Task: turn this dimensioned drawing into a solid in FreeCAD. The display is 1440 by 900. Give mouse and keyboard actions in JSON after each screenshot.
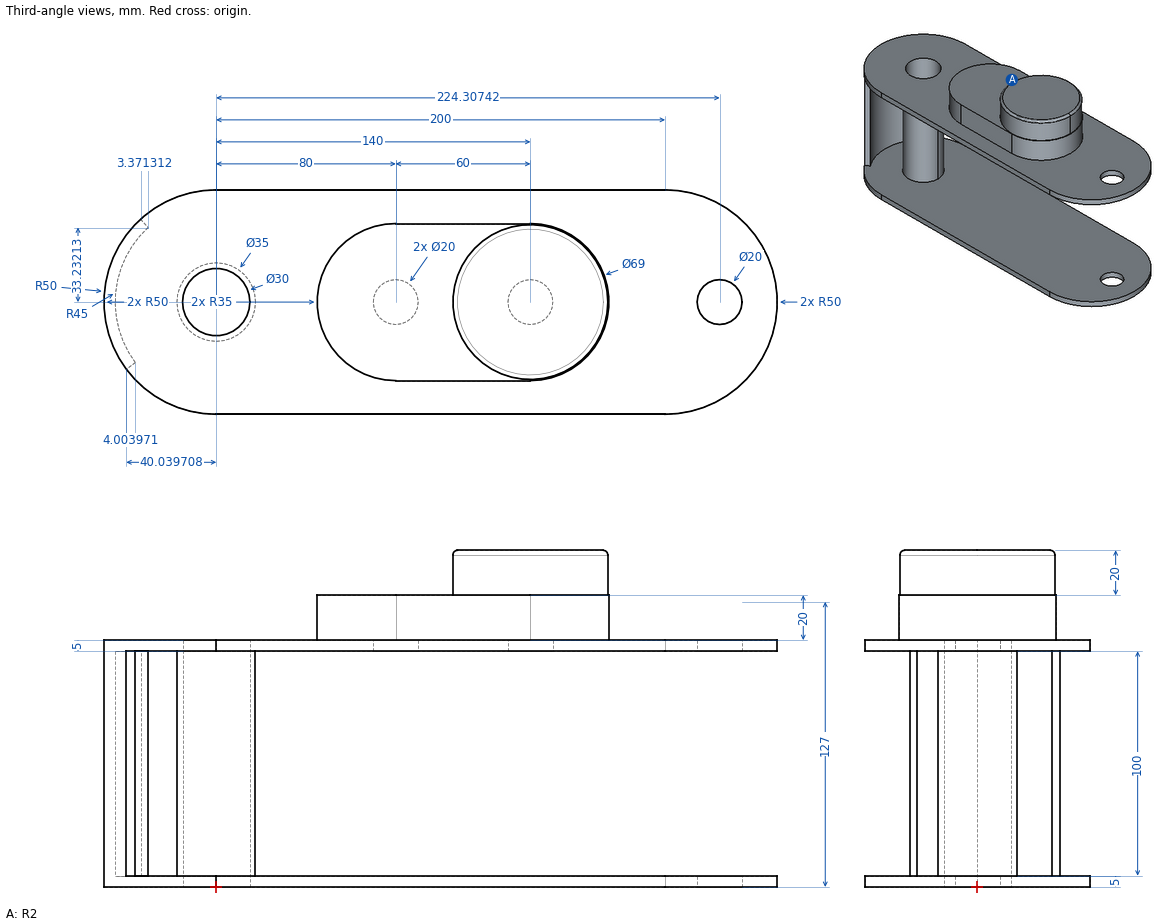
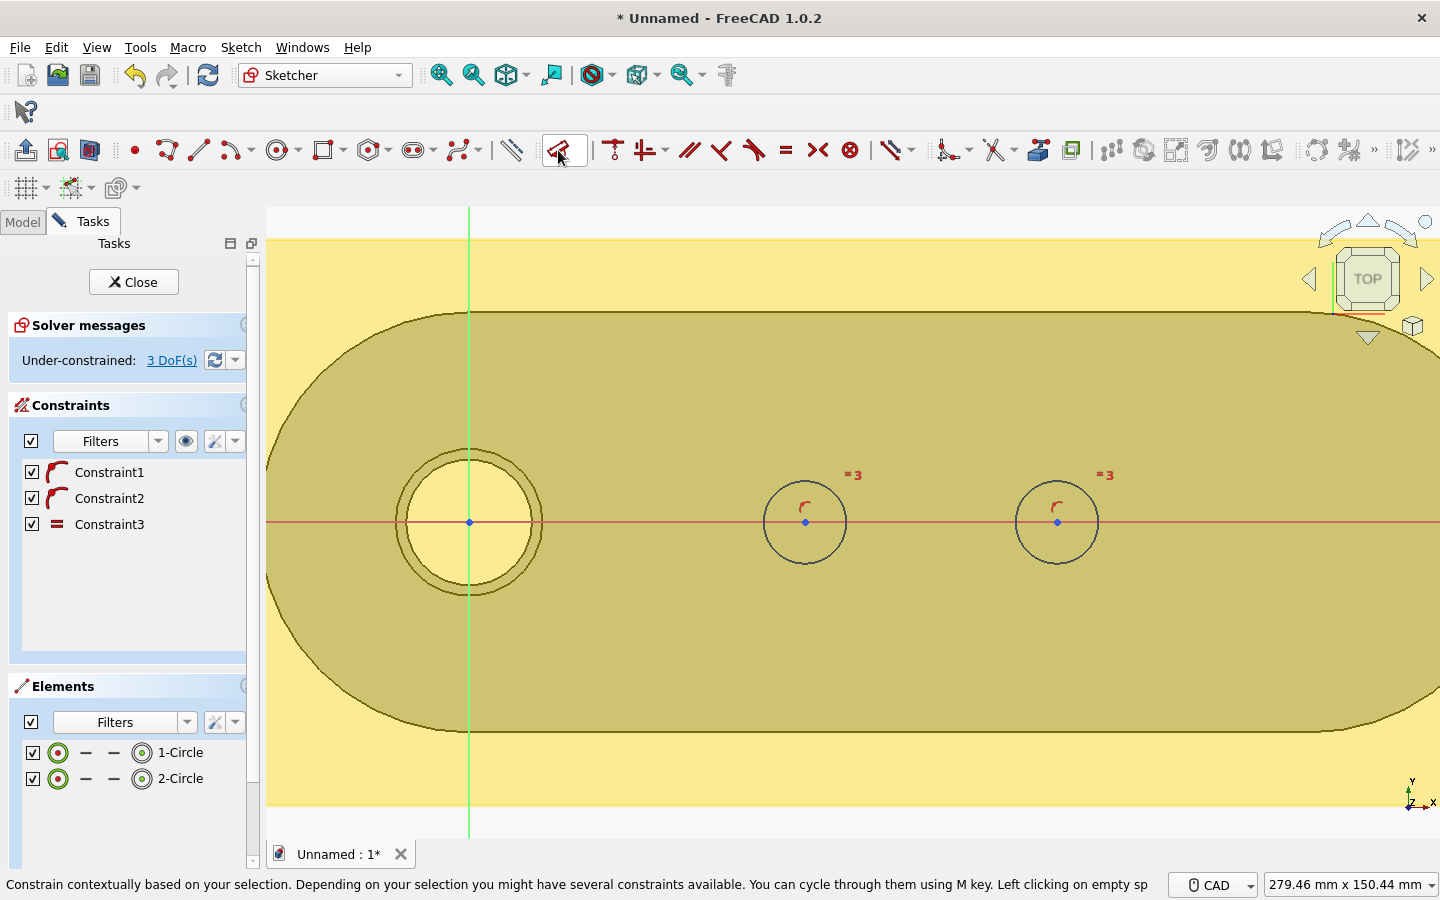
{"action": "left_click", "coordinate": [834, 493]}
{"action": "left_click", "coordinate": [856, 470]}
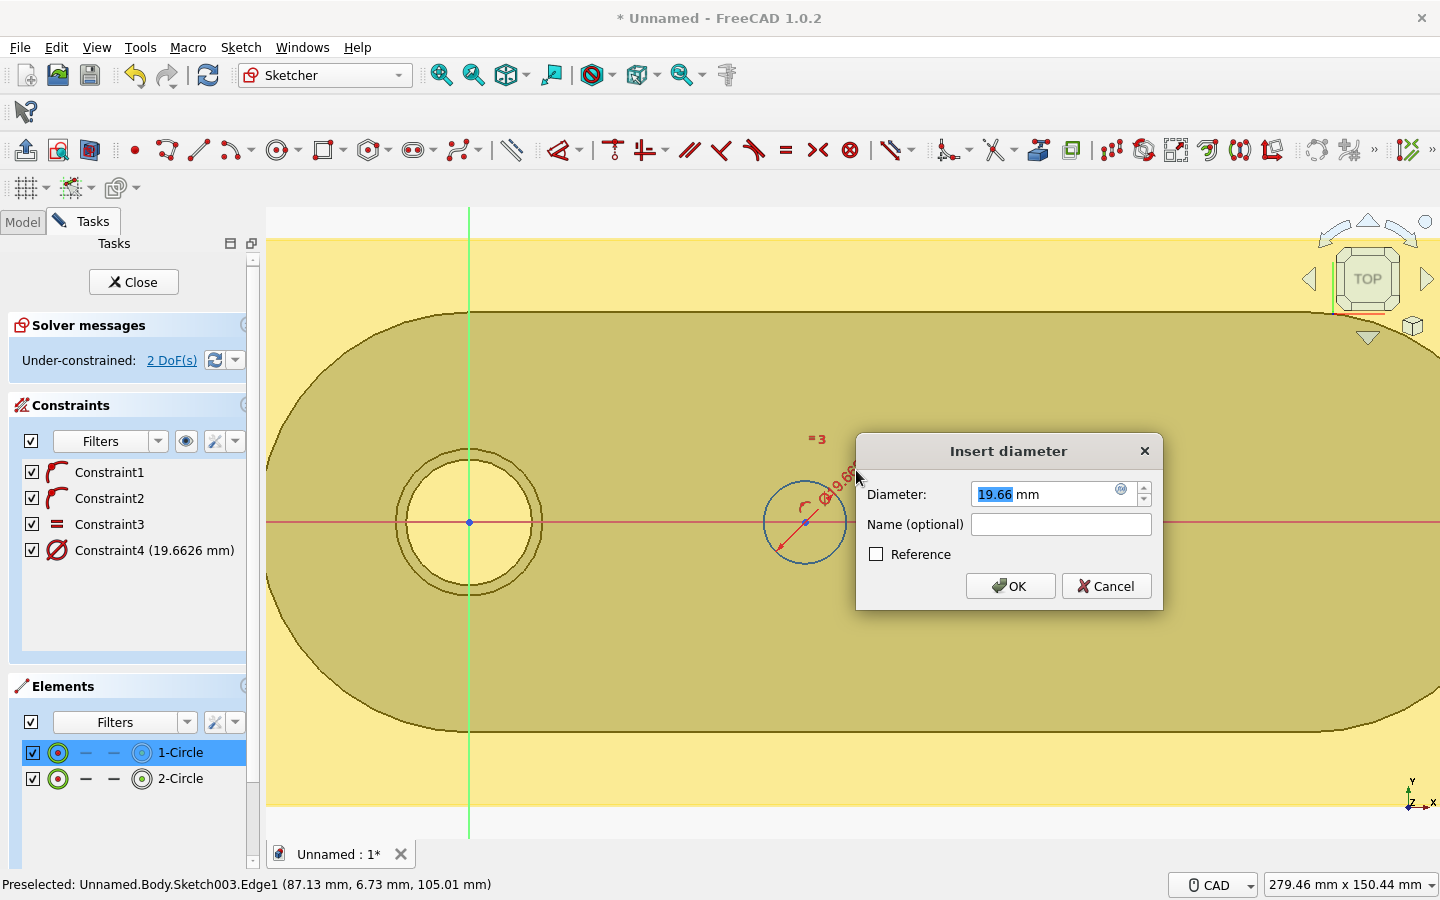
{"action": "type", "text": "20"}
{"action": "key", "text": "Return"}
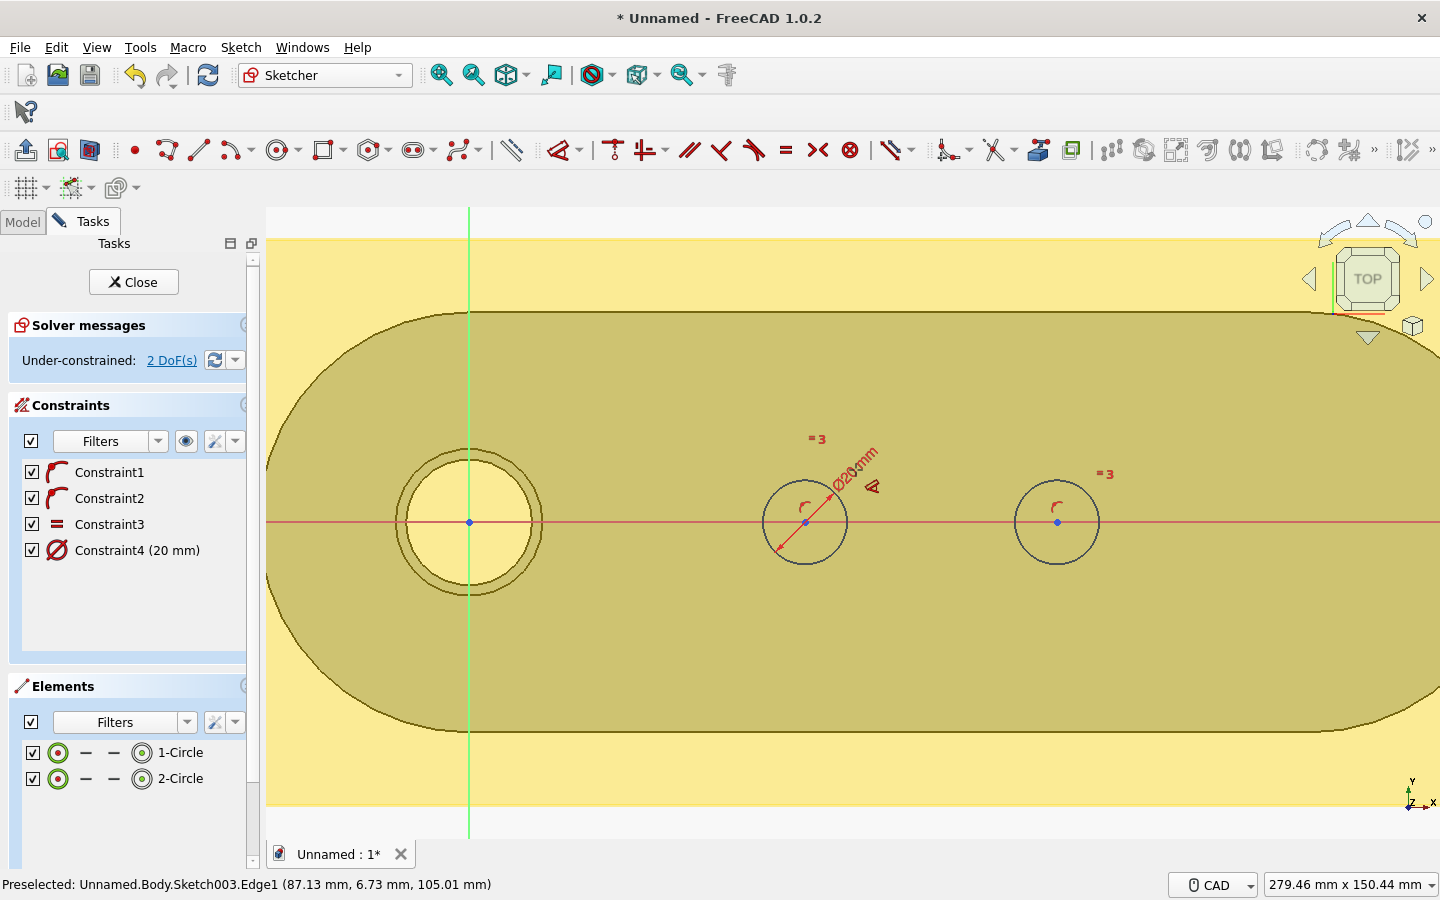
{"action": "left_click", "coordinate": [805, 522]}
{"action": "left_click", "coordinate": [637, 556]}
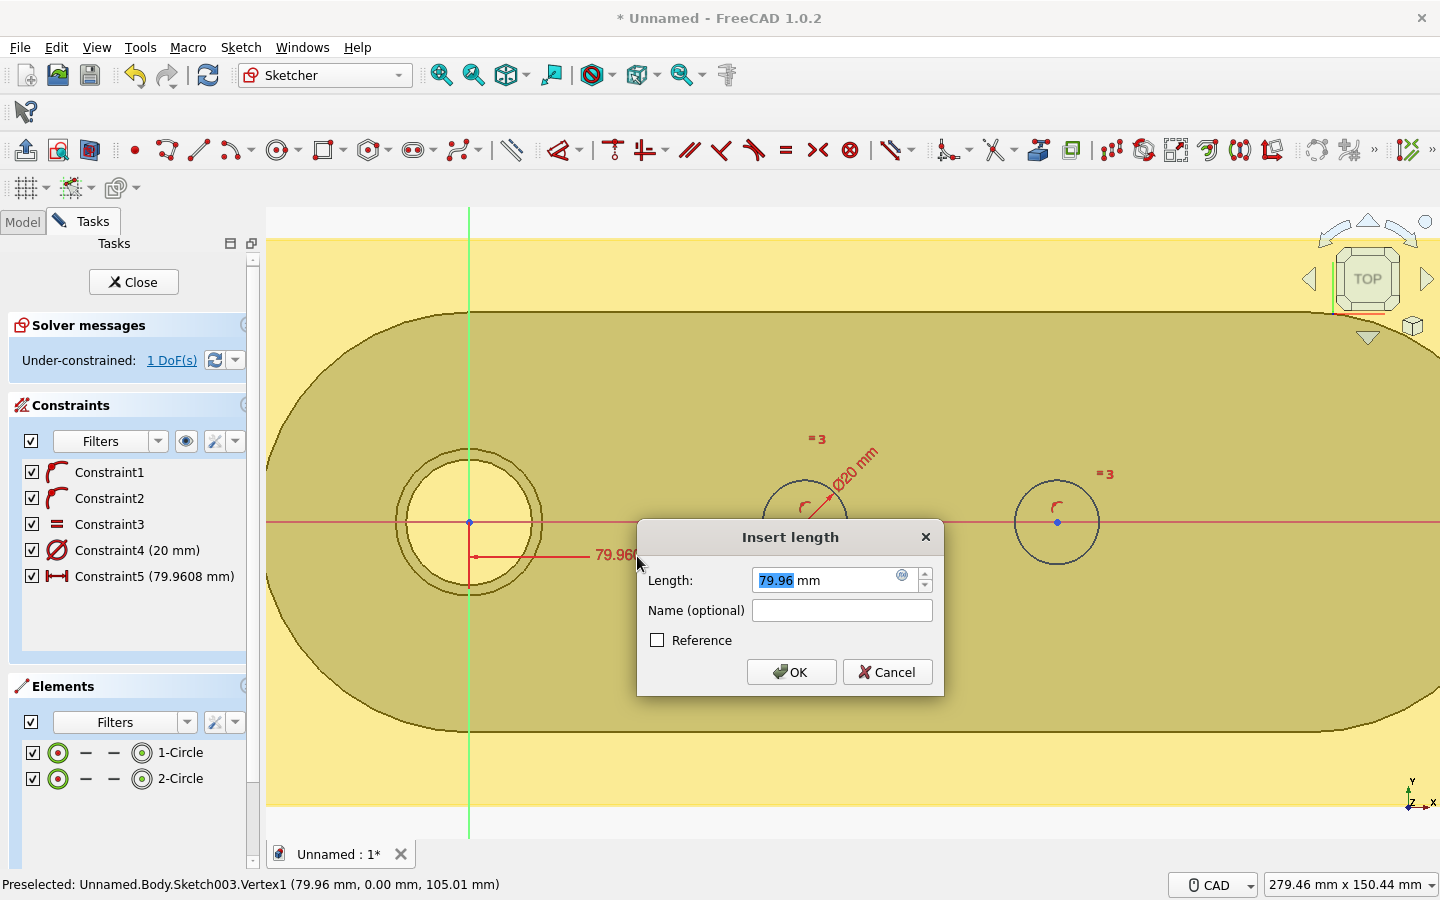
{"action": "type", "text": "80"}
{"action": "key", "text": "Return"}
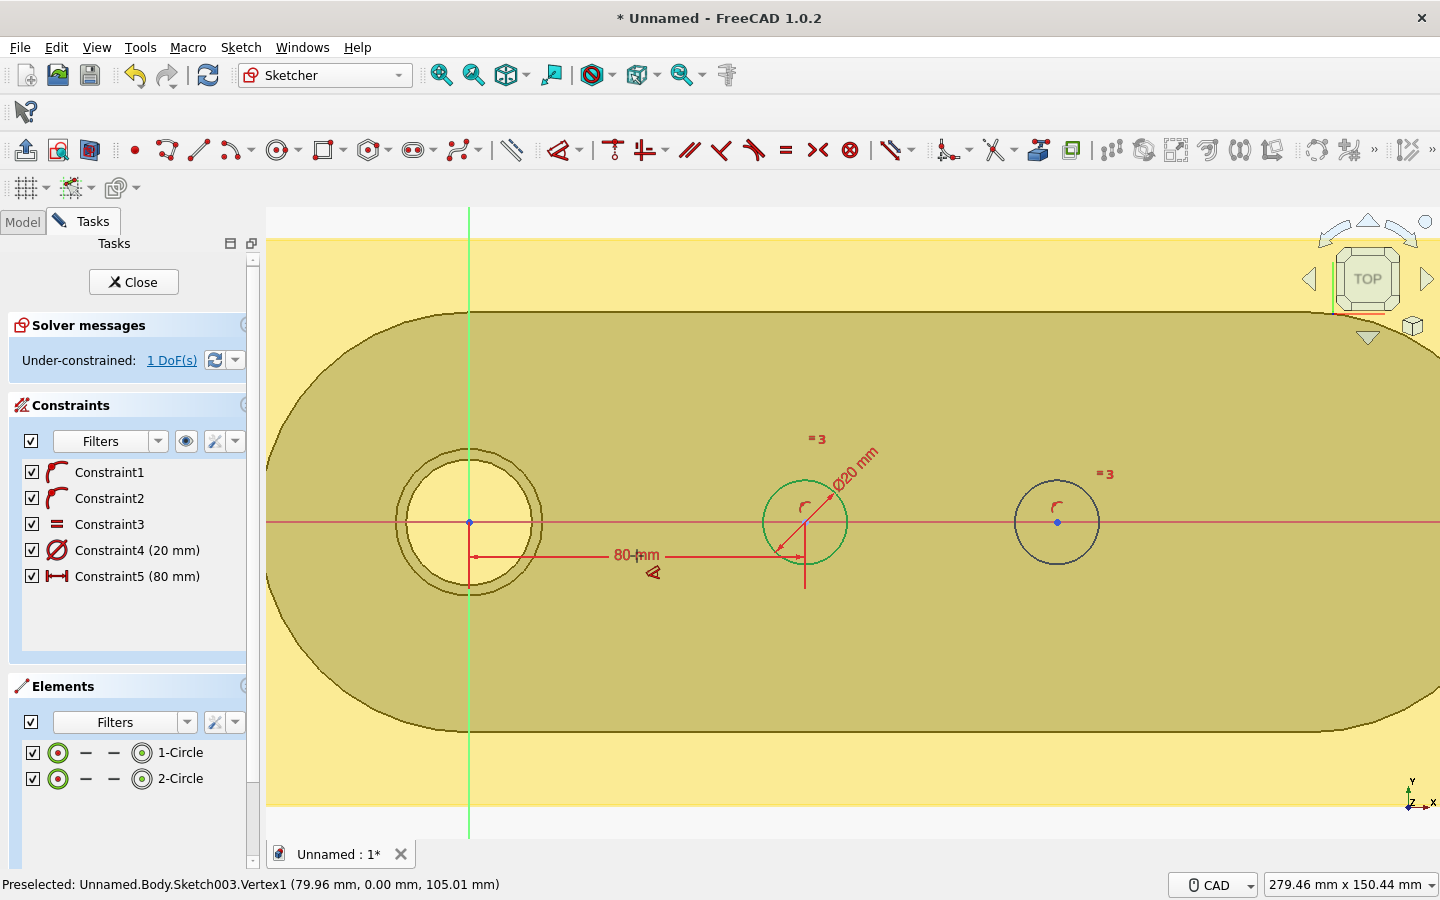
{"action": "left_click", "coordinate": [1057, 522]}
{"action": "left_click", "coordinate": [898, 556]}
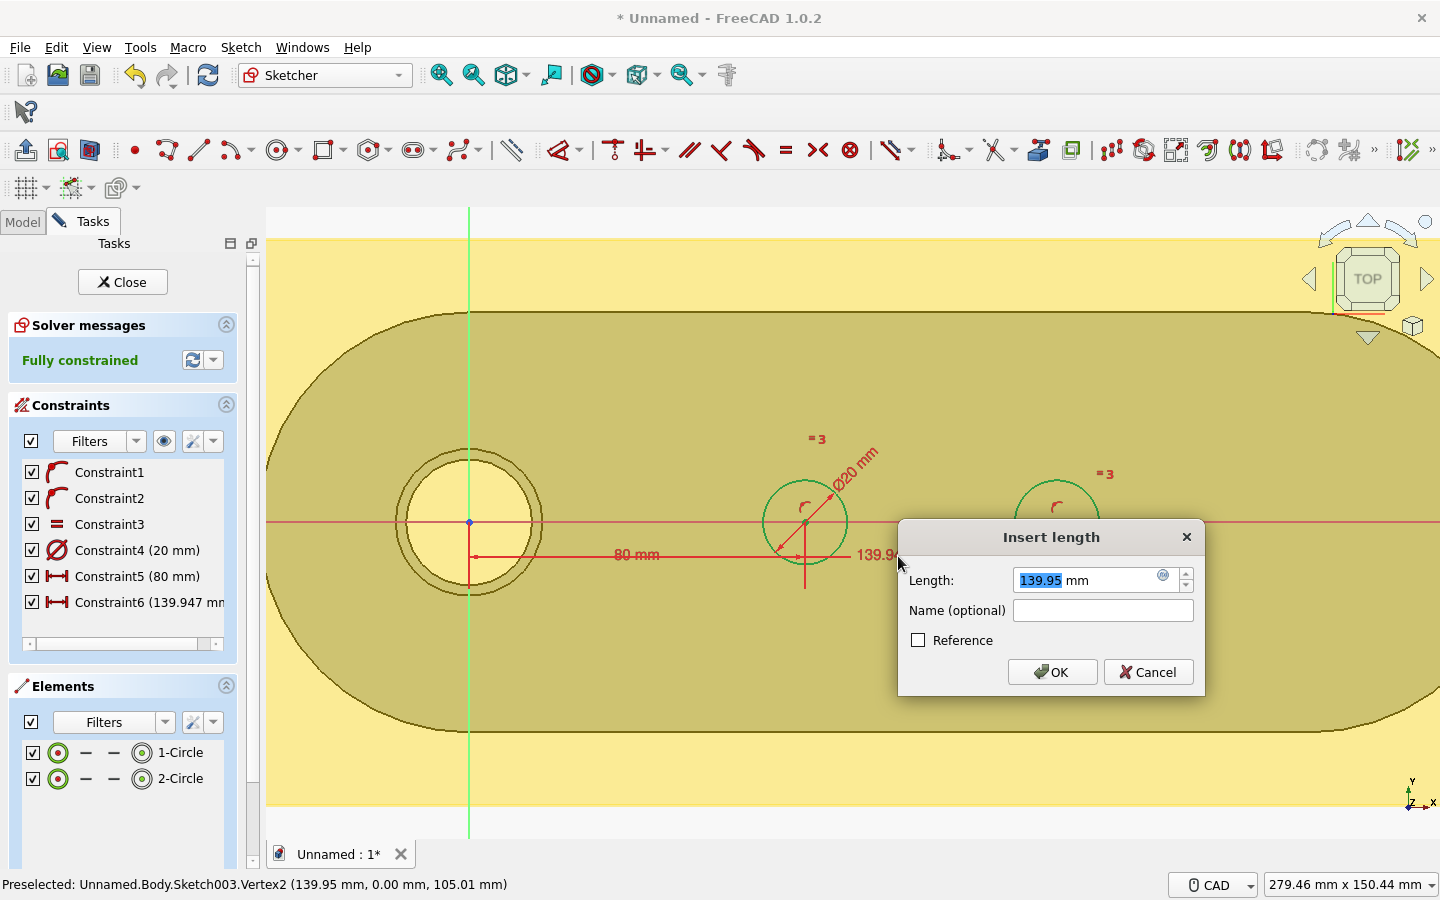
{"action": "type", "text": "140"}
{"action": "key", "text": "Return"}
{"action": "key", "text": "Escape"}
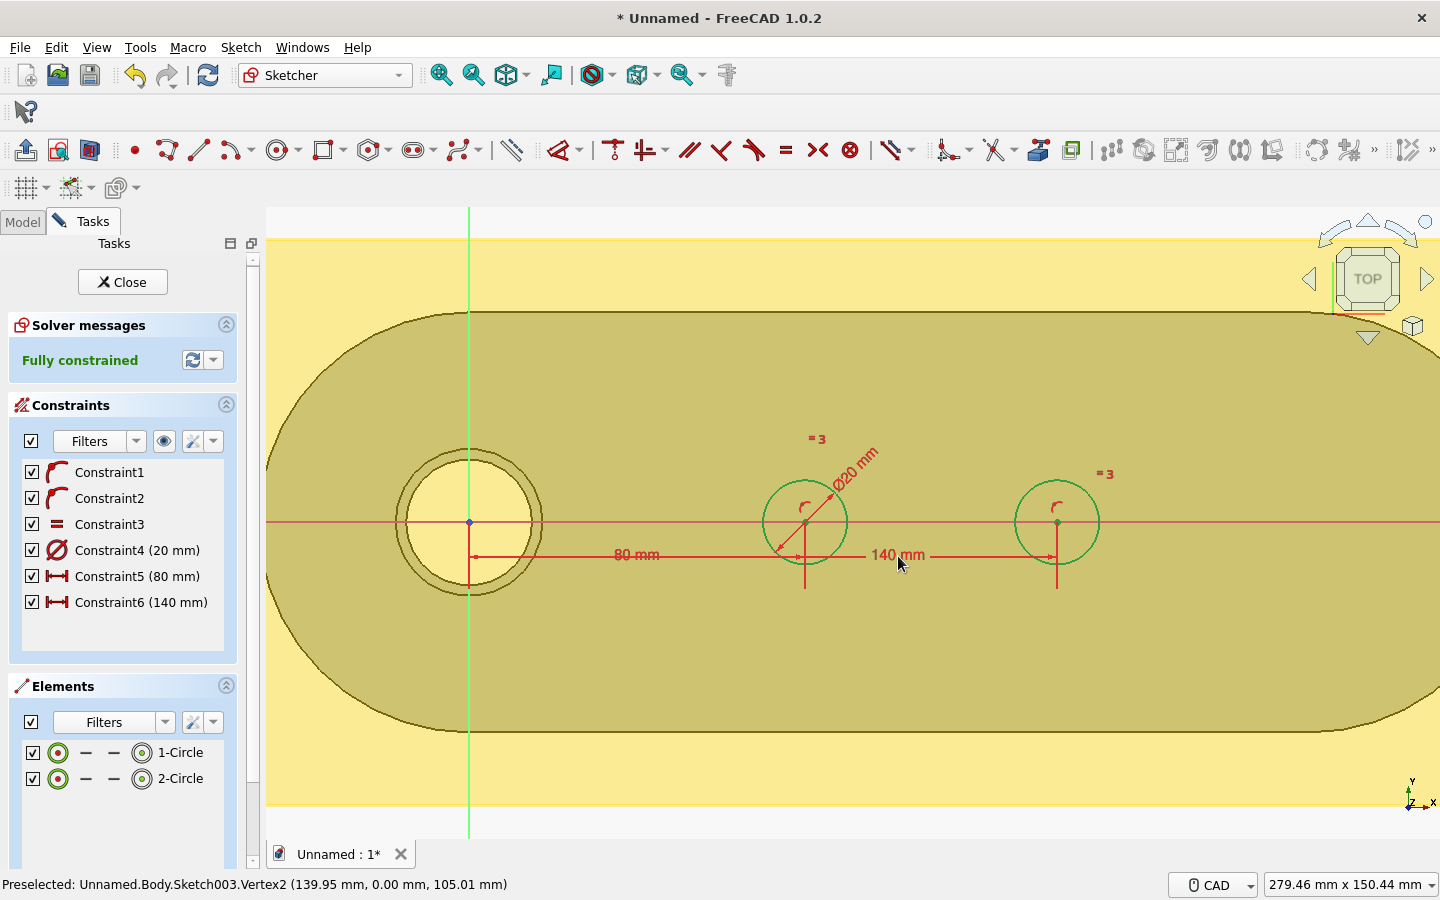
{"action": "left_click", "coordinate": [123, 282]}